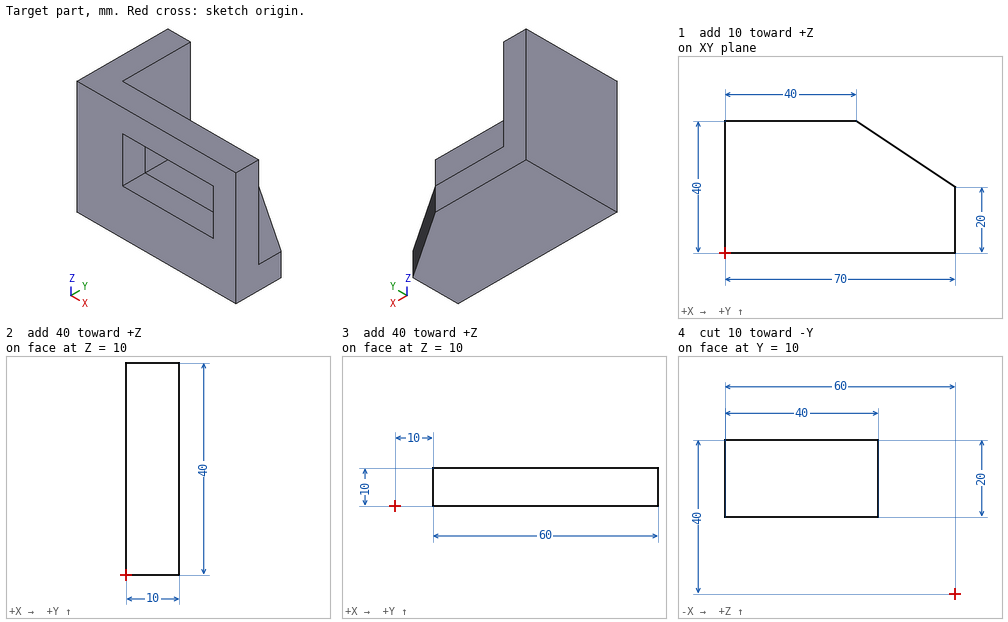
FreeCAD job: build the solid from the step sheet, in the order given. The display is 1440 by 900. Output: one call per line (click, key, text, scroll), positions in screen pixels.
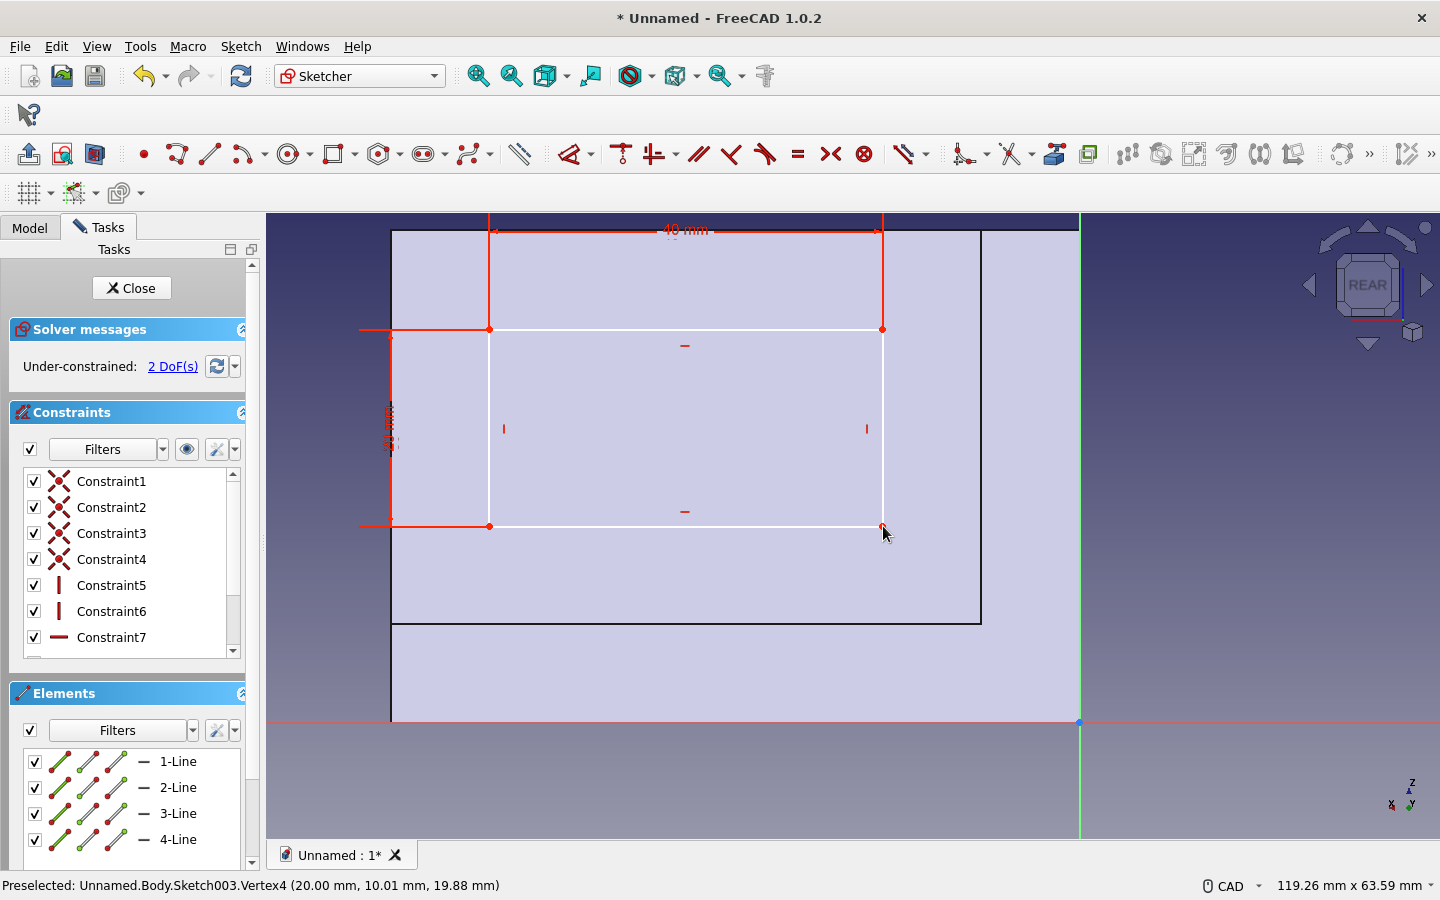
key(d)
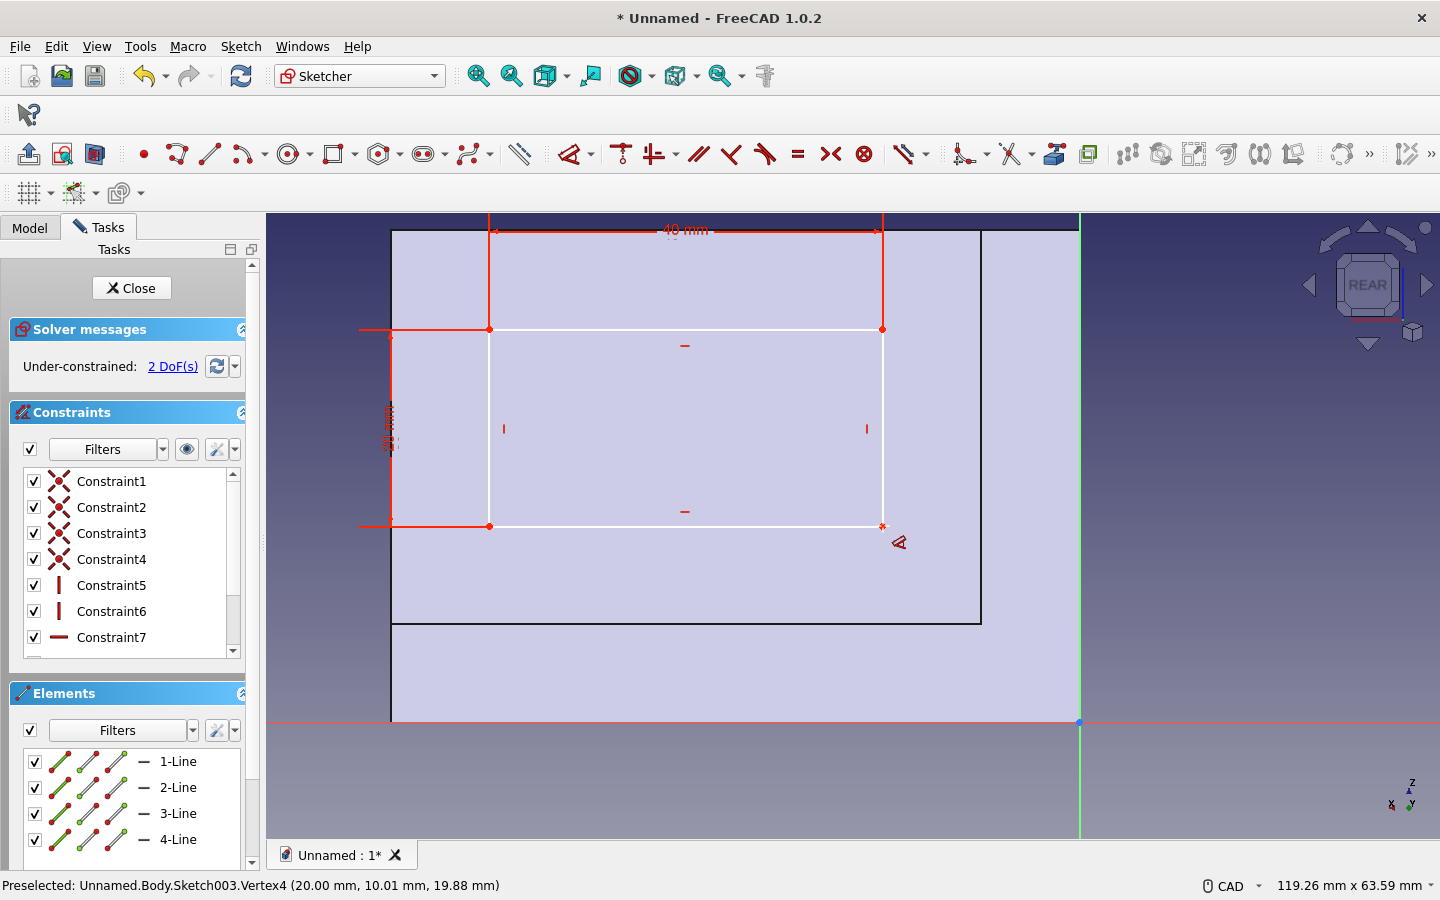
click(489, 330)
click(784, 757)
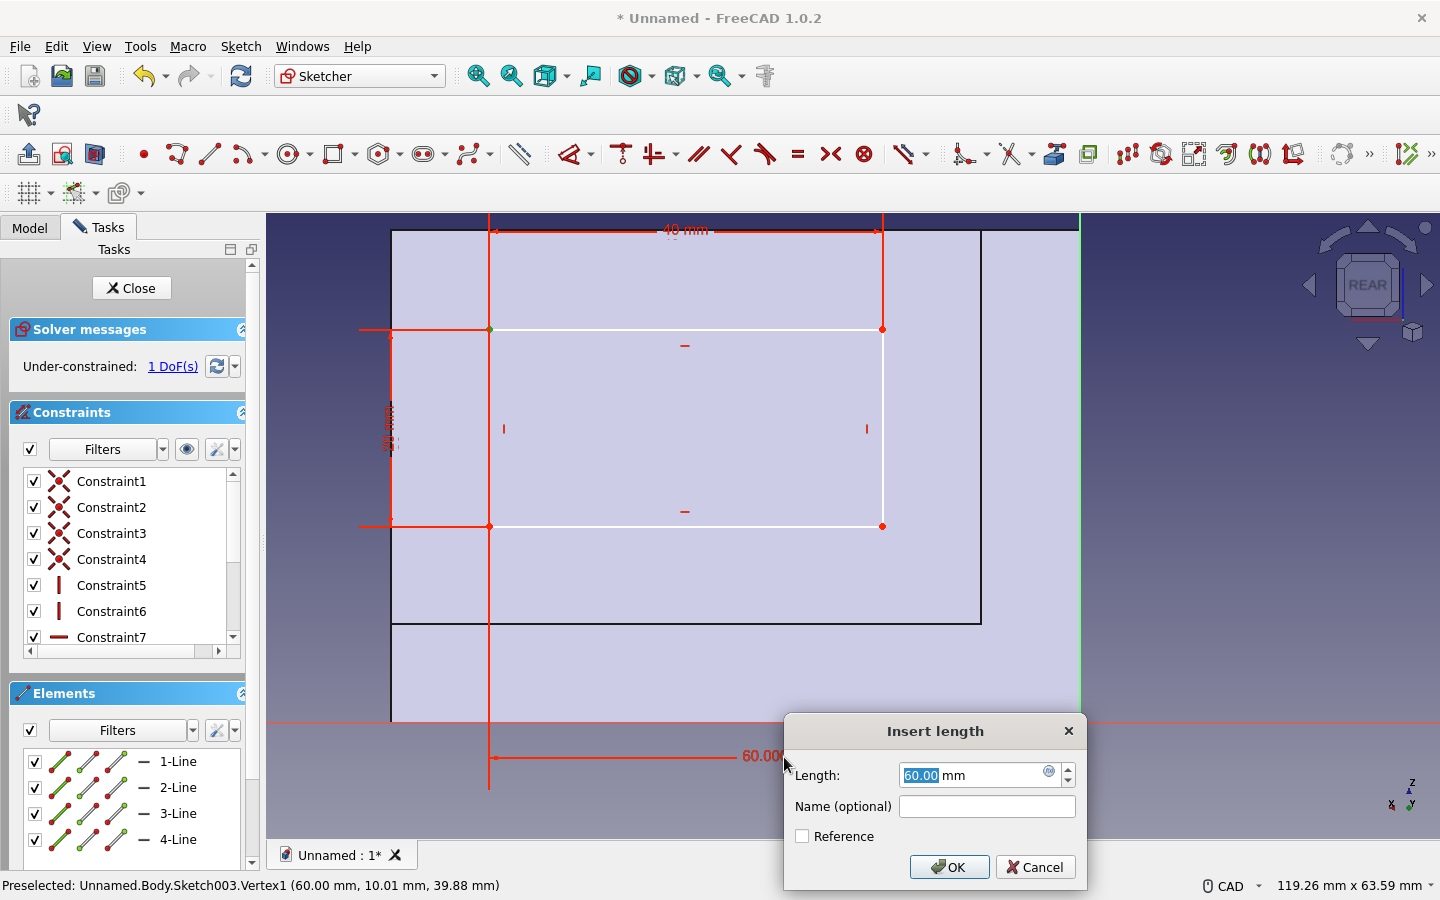
text(60)
key(Return)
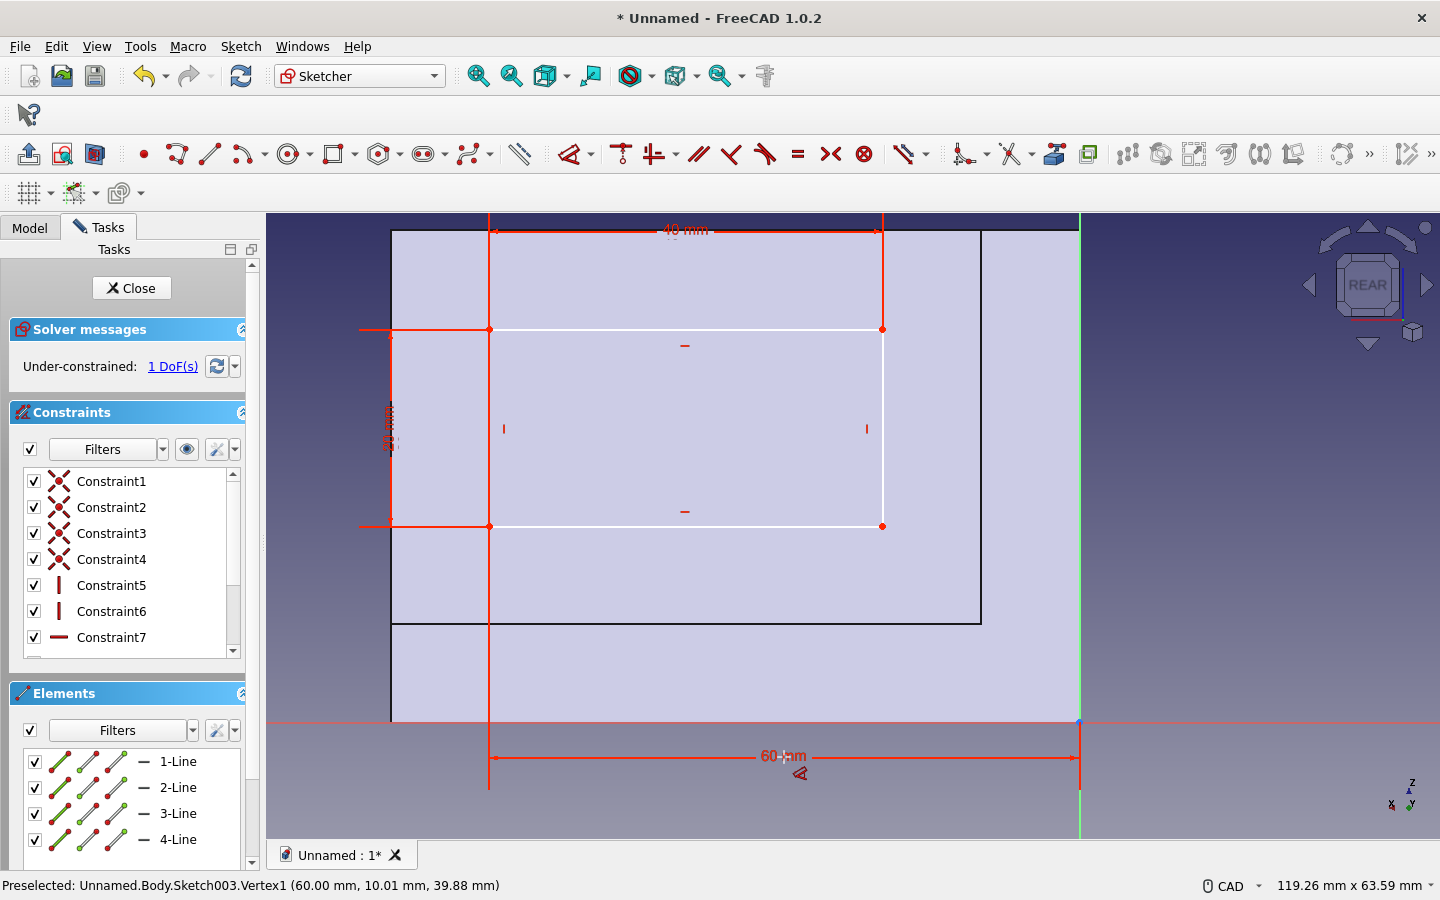
click(489, 330)
click(1114, 526)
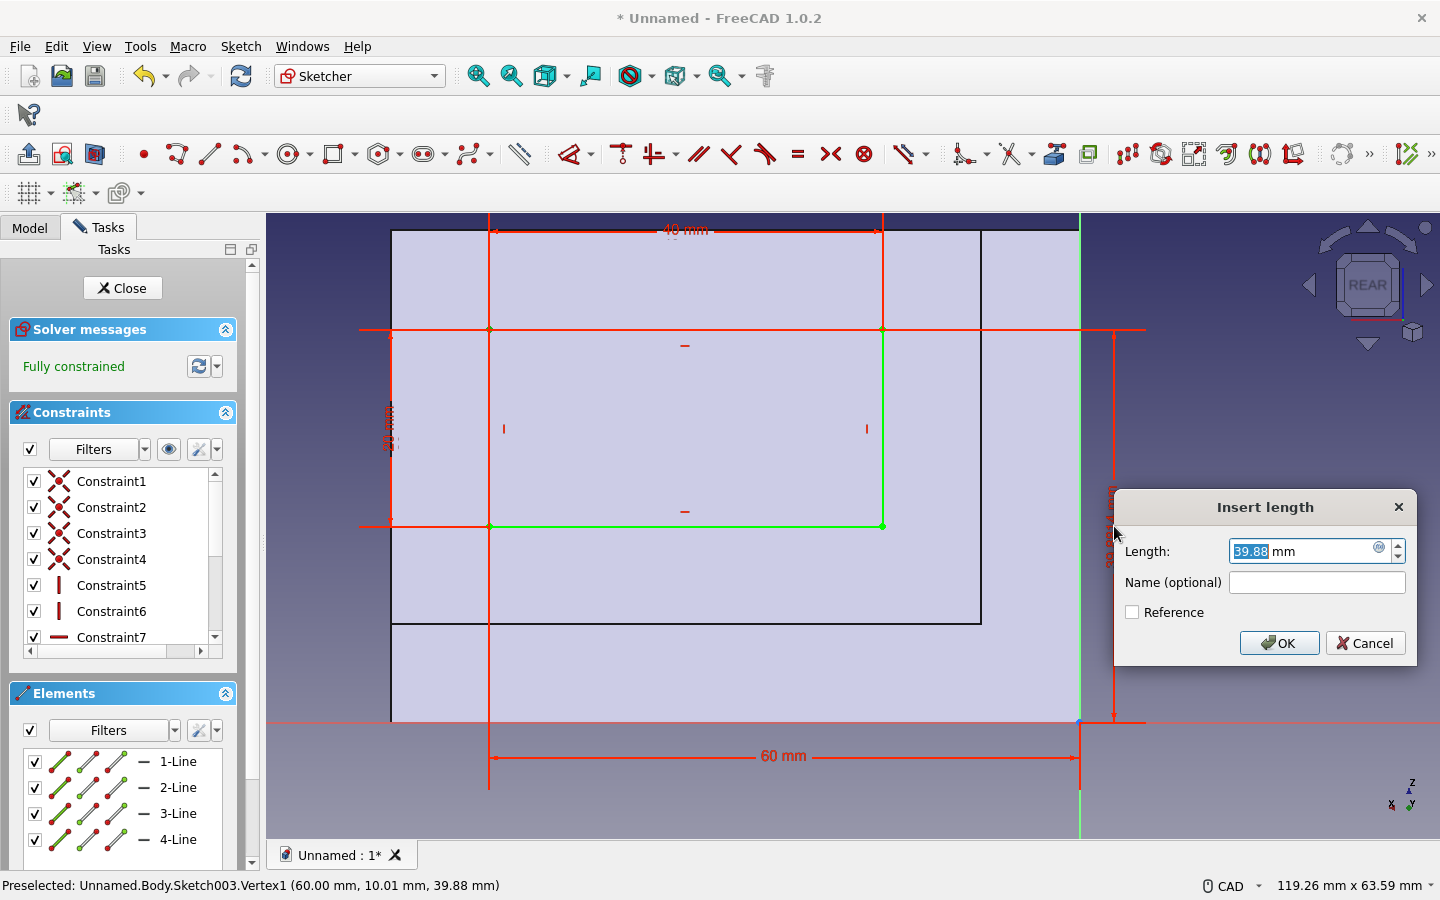
text(40)
key(Return)
key(Escape)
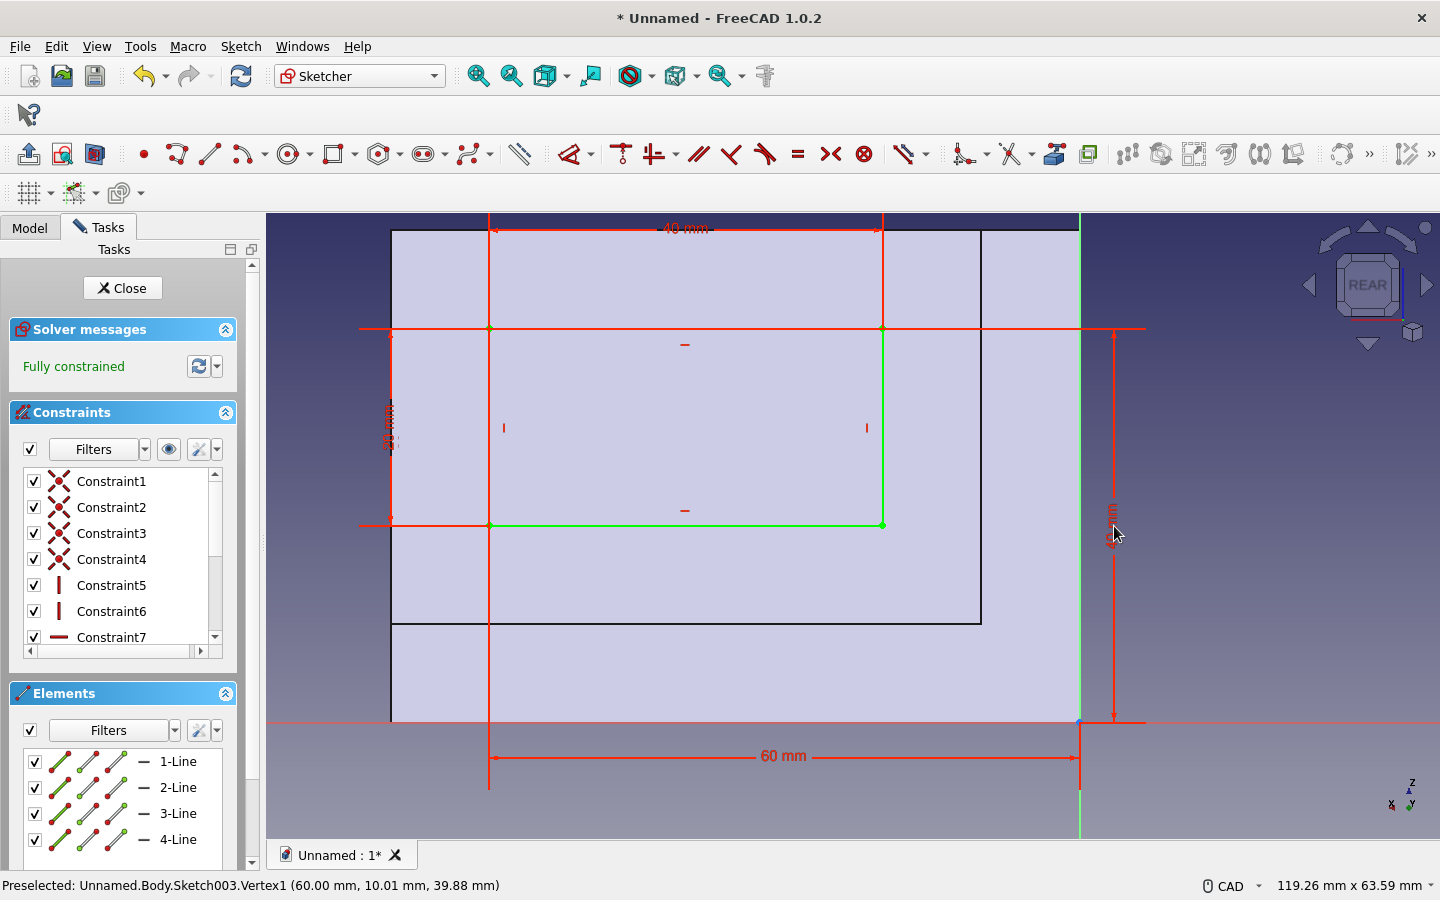
click(123, 288)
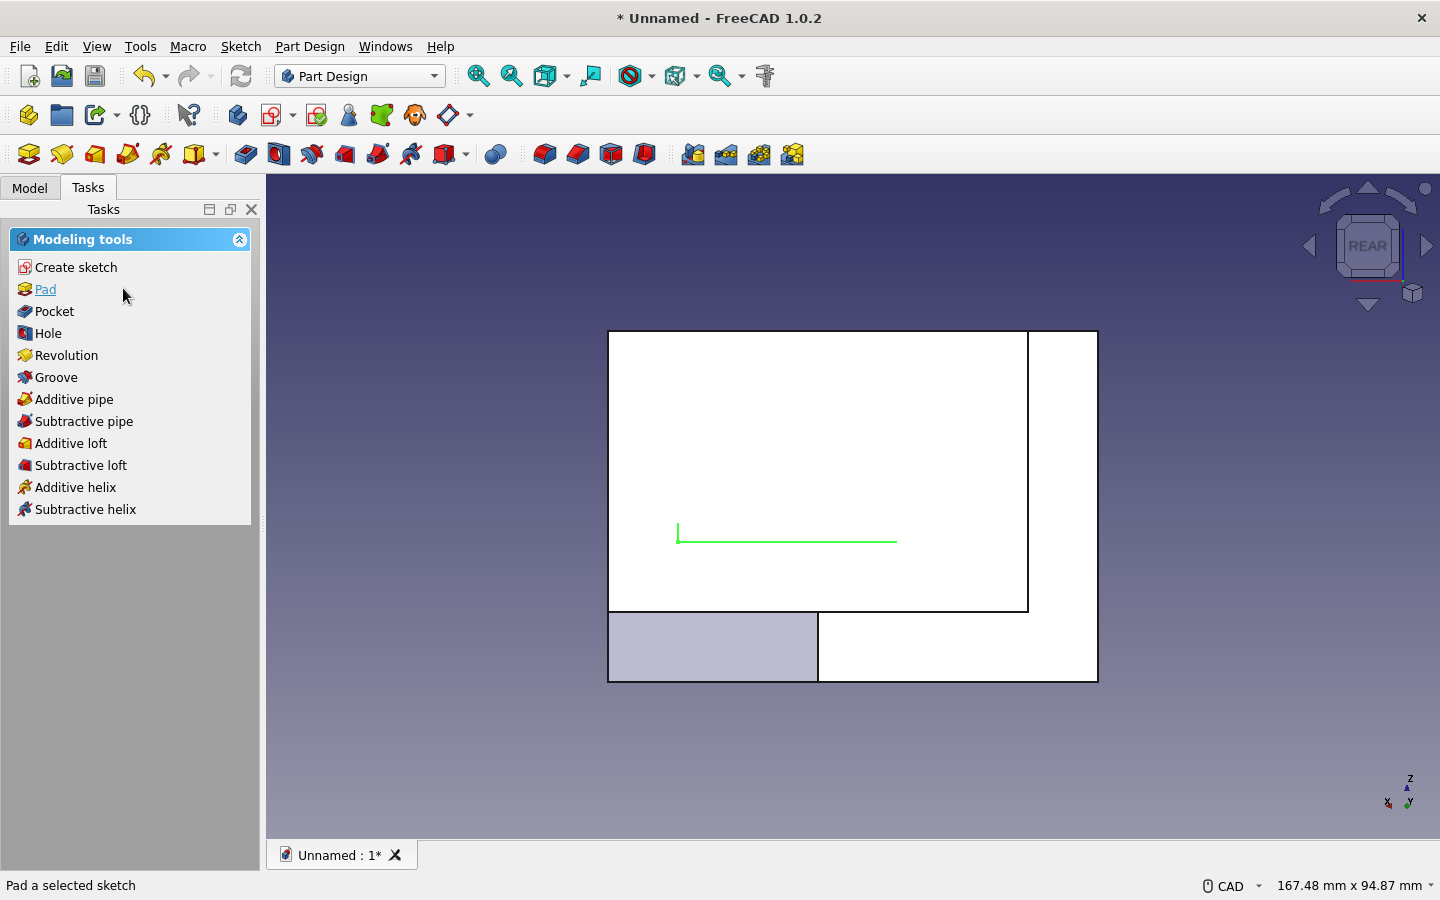
click(246, 154)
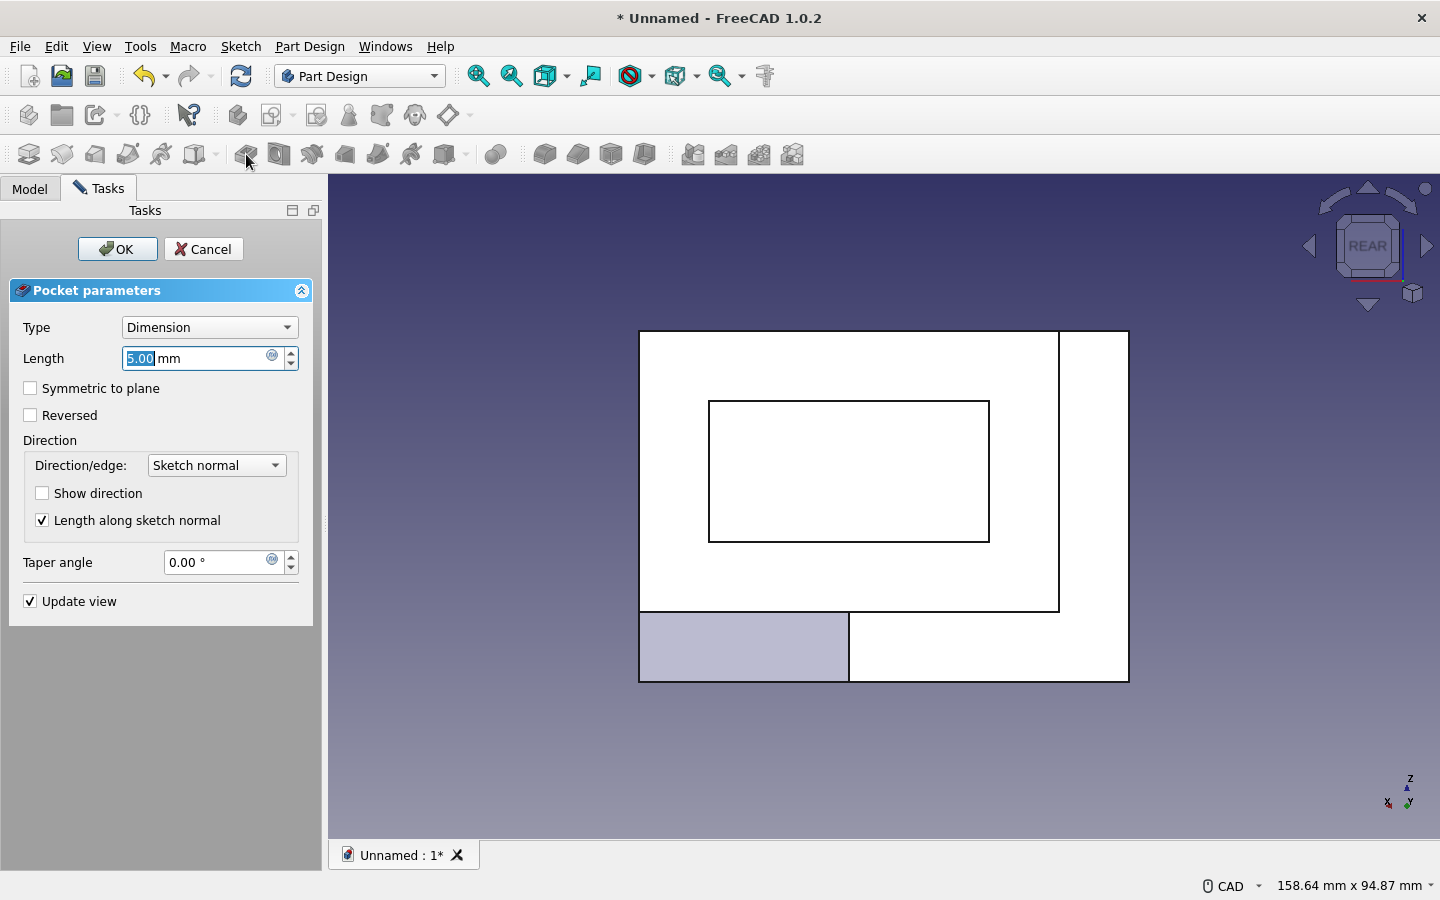
text(10)
key(Tab)